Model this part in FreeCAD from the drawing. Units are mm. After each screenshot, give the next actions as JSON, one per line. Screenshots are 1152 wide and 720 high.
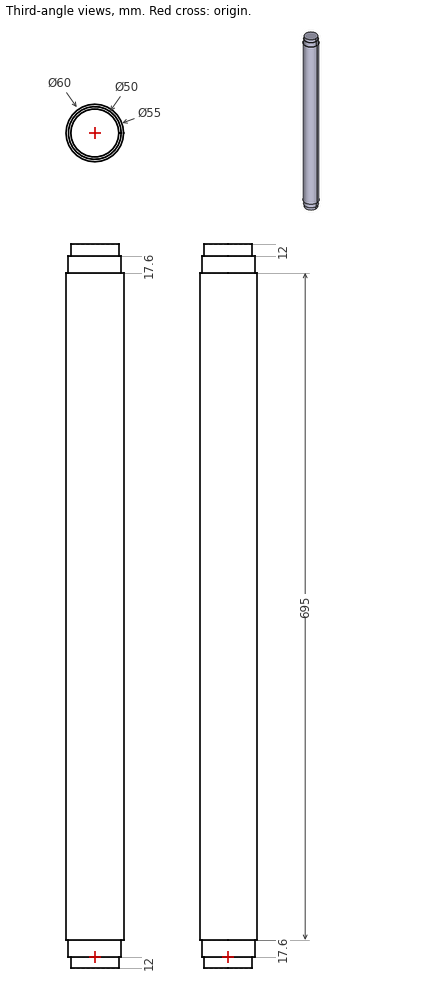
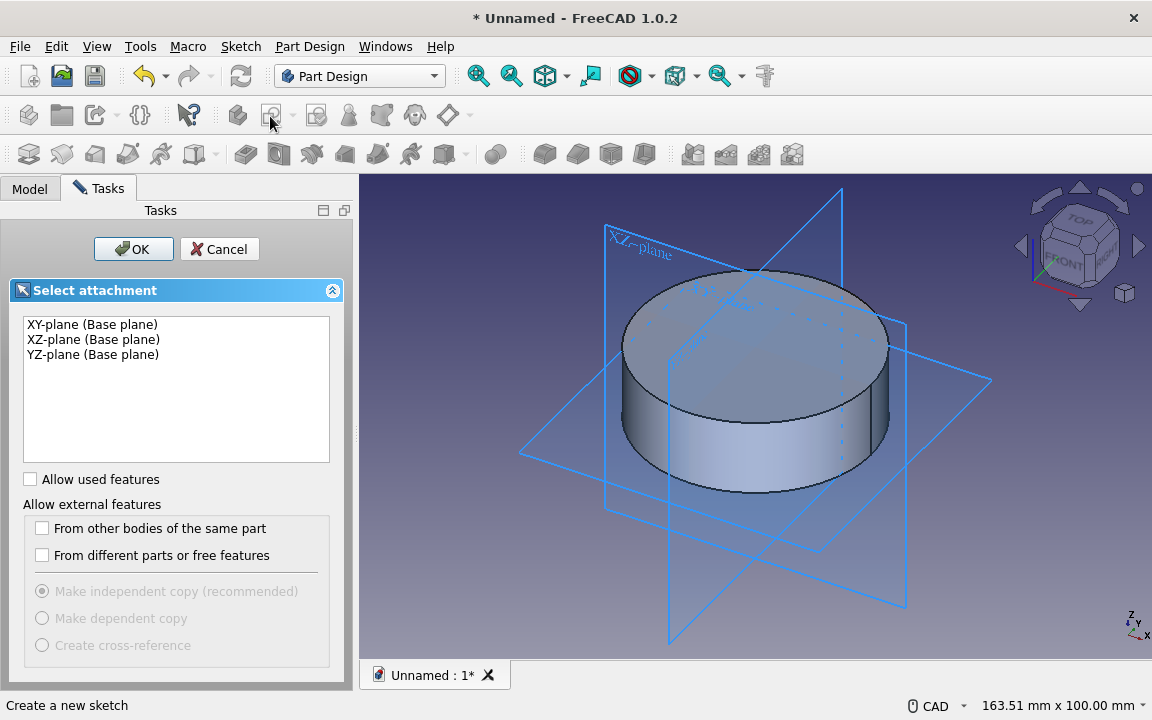
{"action": "left_click", "coordinate": [84, 324]}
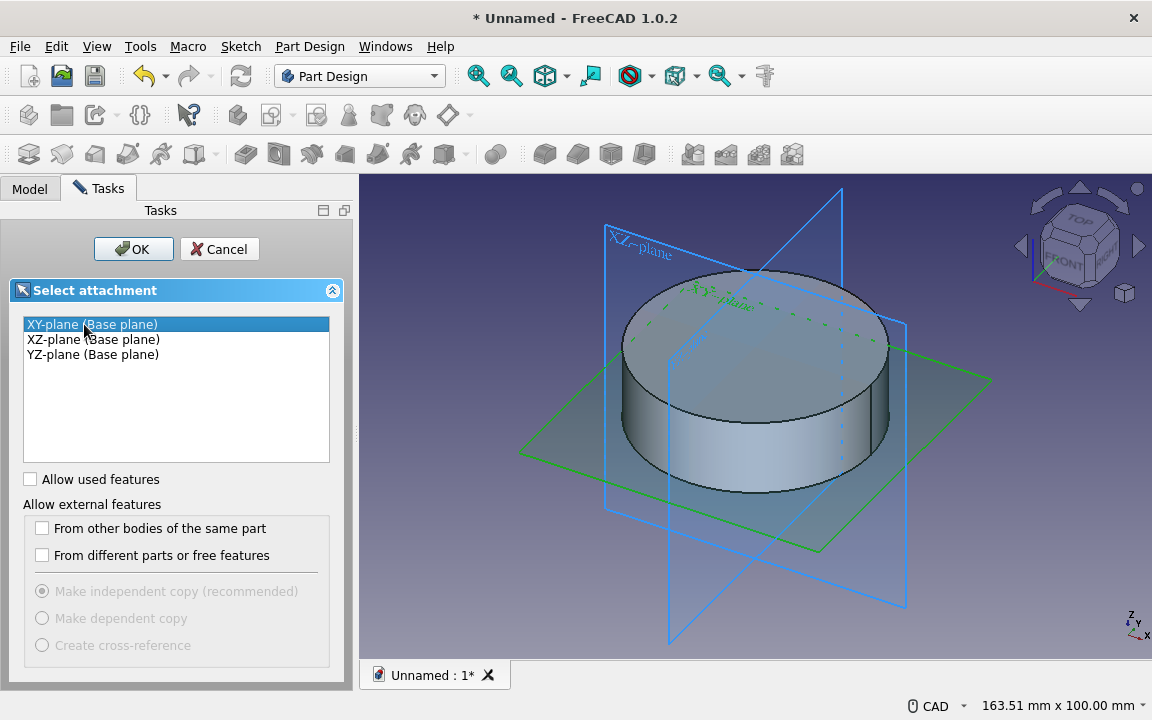
{"action": "left_click", "coordinate": [134, 249]}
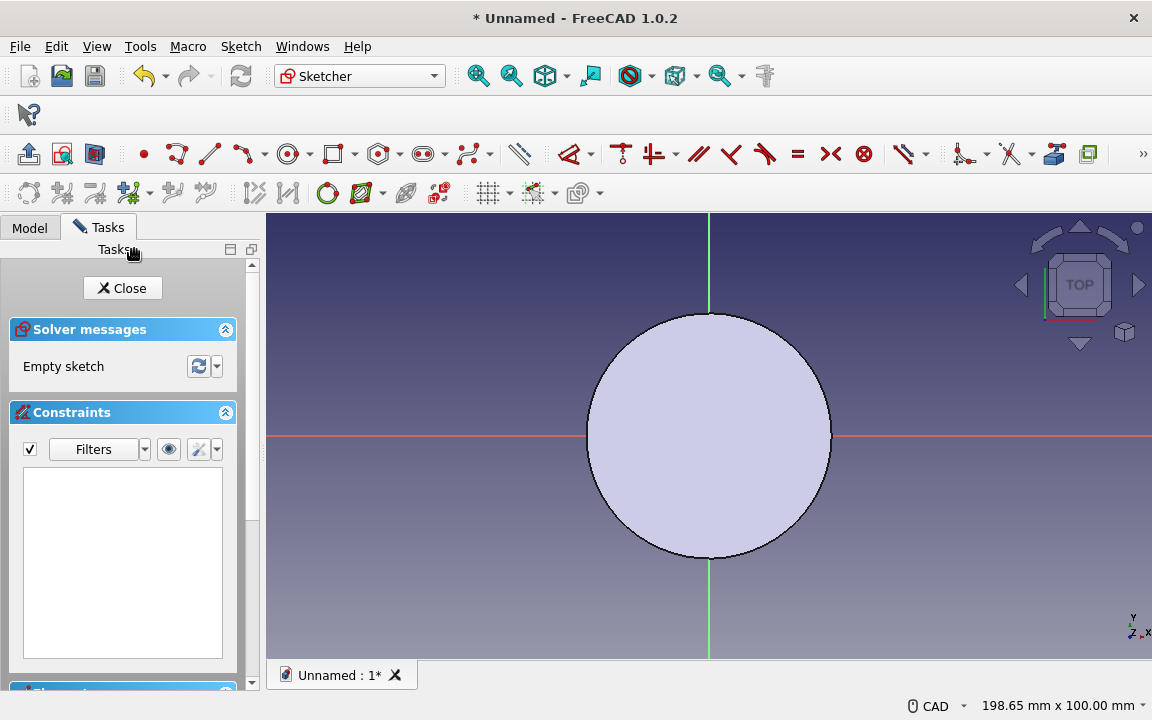
{"action": "left_click", "coordinate": [95, 154]}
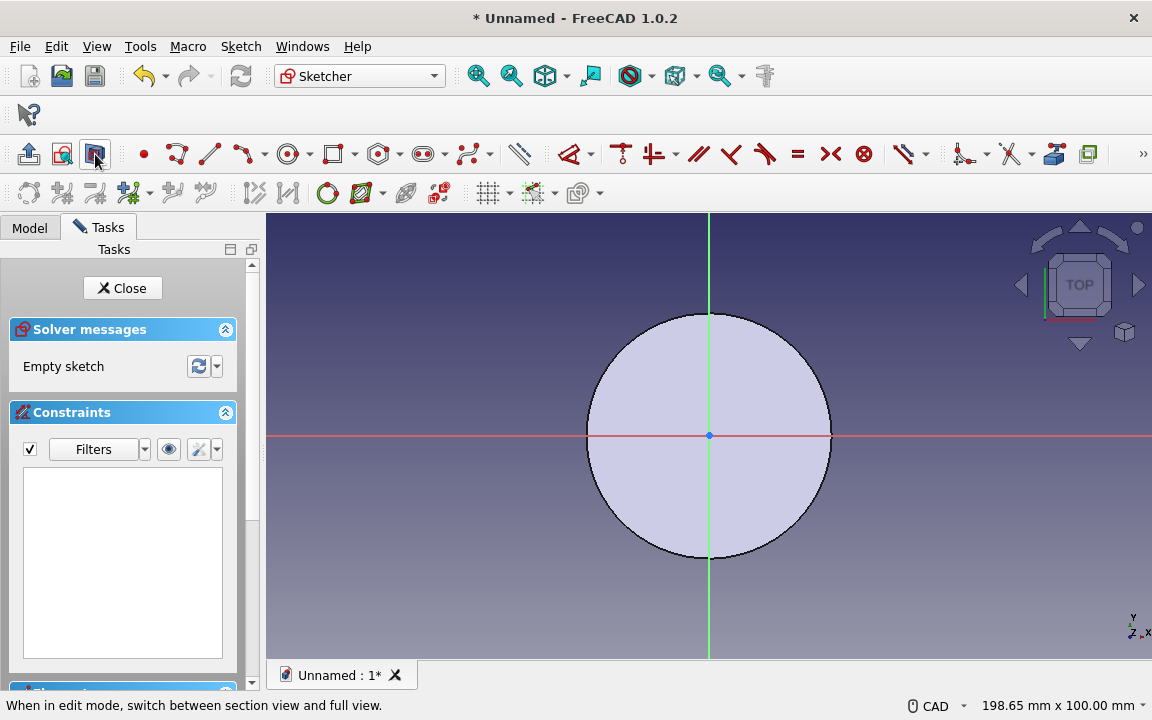
{"action": "left_click", "coordinate": [288, 154]}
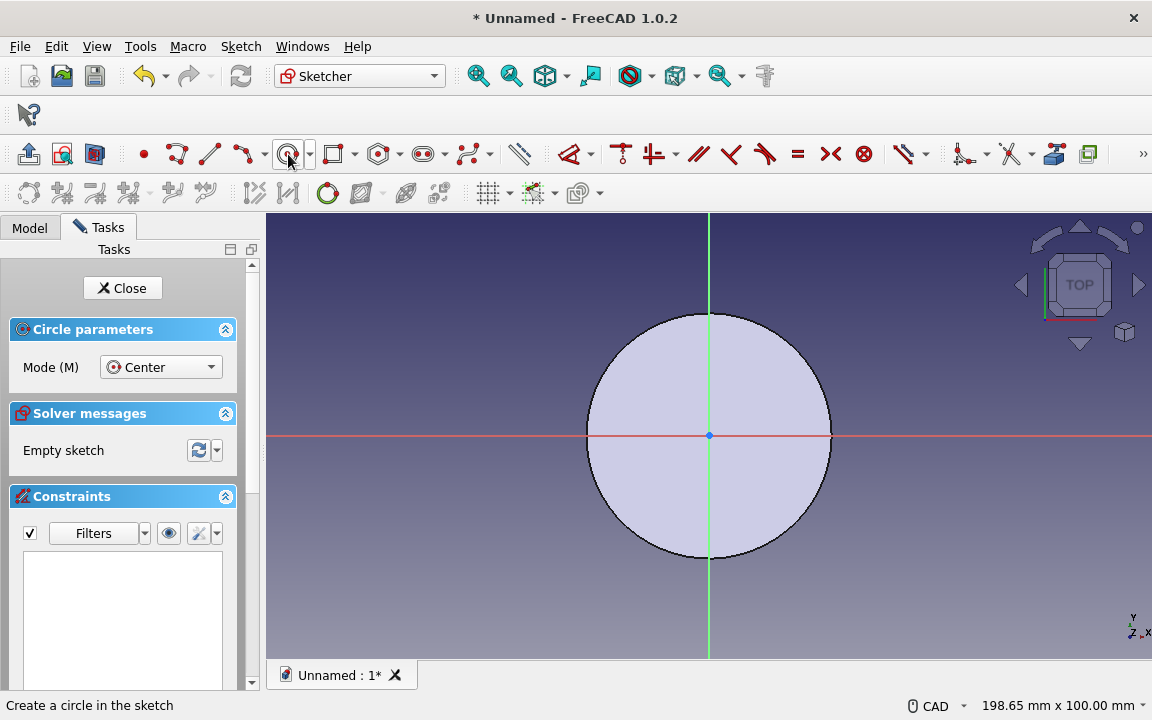
{"action": "left_click", "coordinate": [709, 436]}
{"action": "mouse_move", "coordinate": [788, 357]}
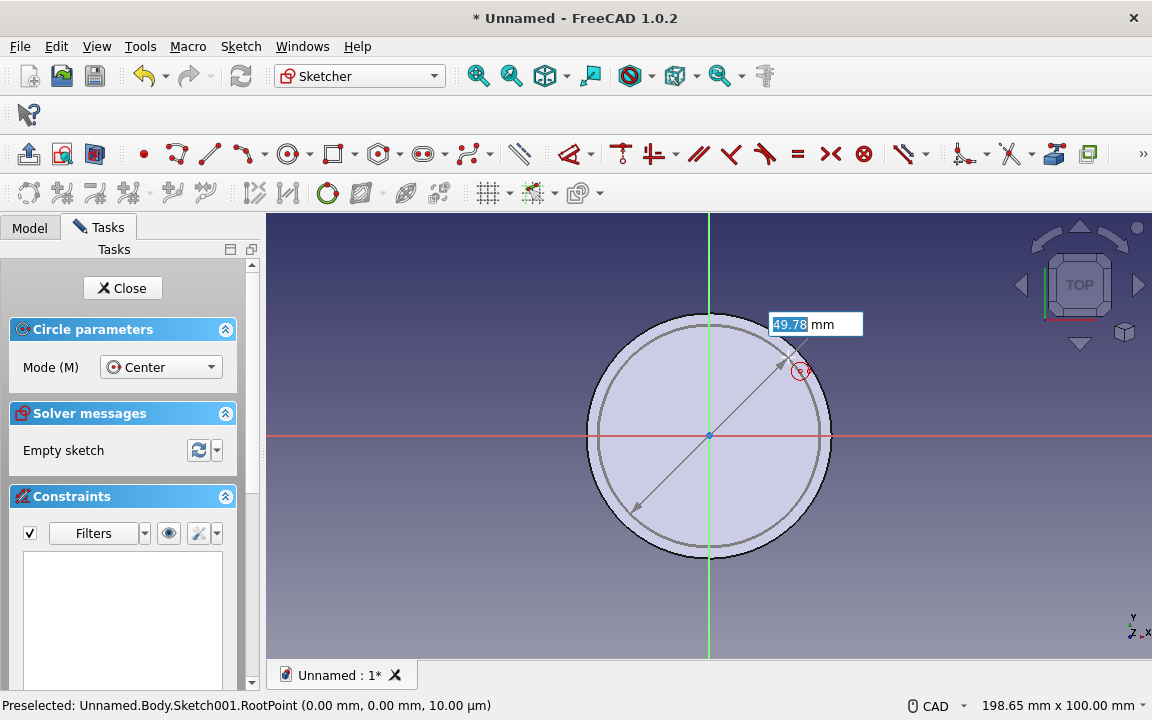
{"action": "type", "text": "50"}
{"action": "key", "text": "Return"}
{"action": "key", "text": "Escape"}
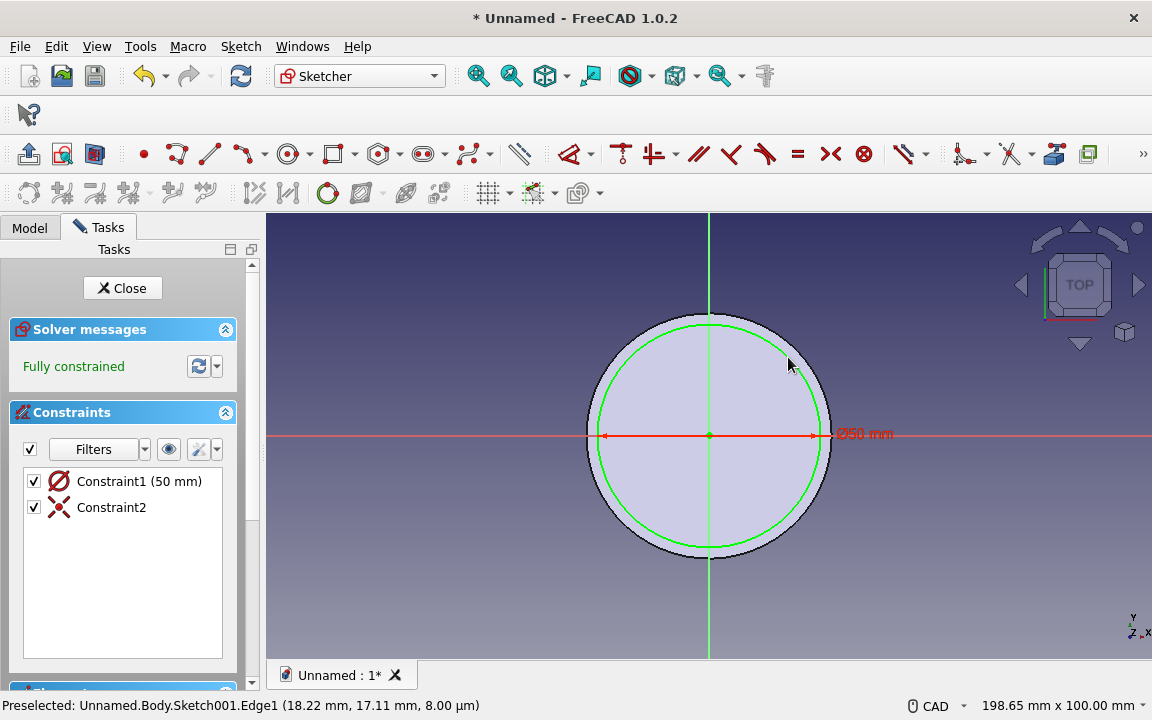
{"action": "left_click", "coordinate": [123, 288]}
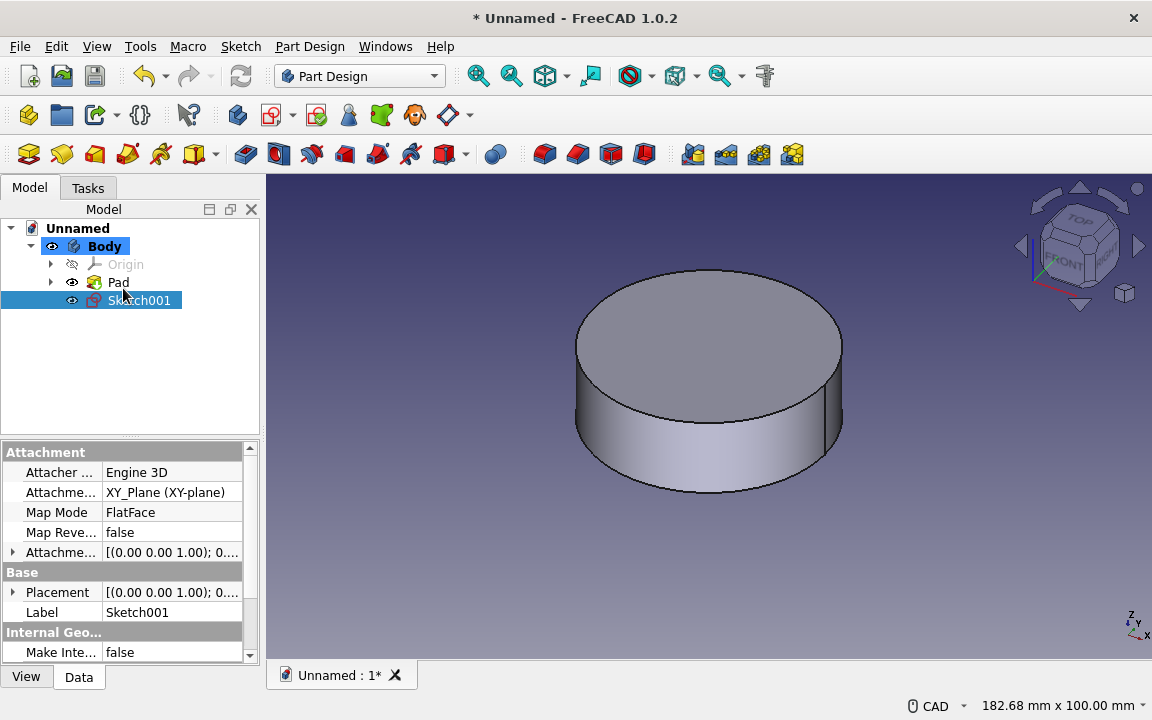
{"action": "left_click", "coordinate": [29, 154]}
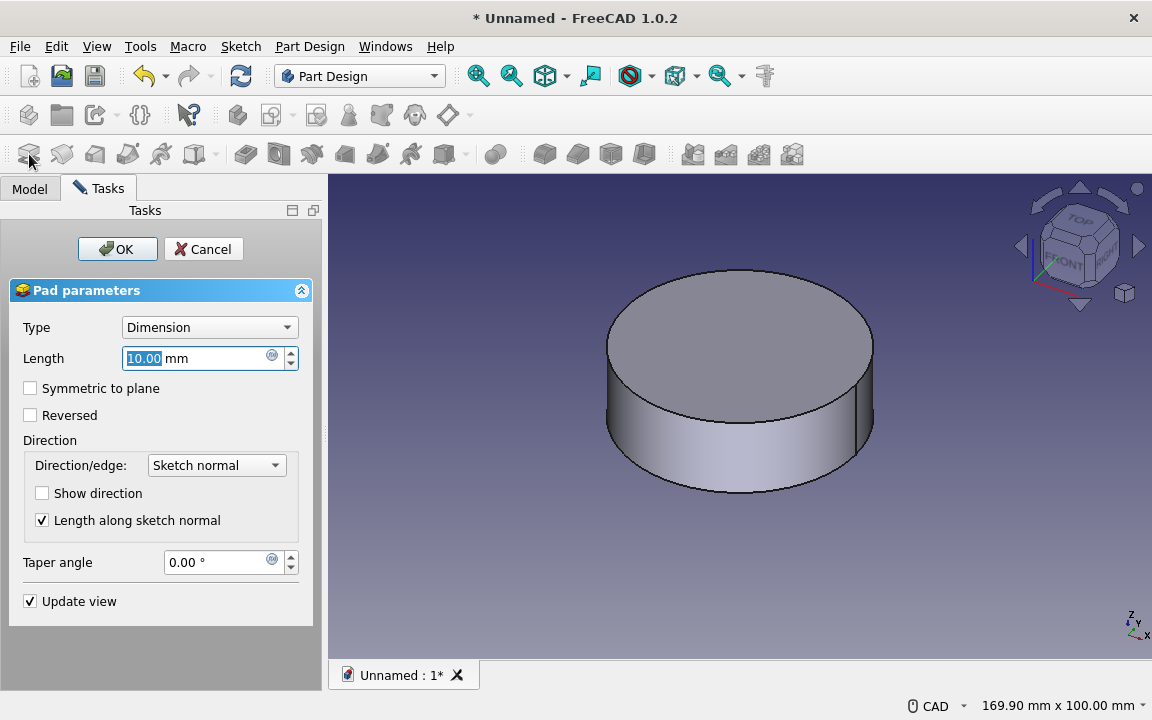
{"action": "type", "text": "12"}
{"action": "key", "text": "Tab"}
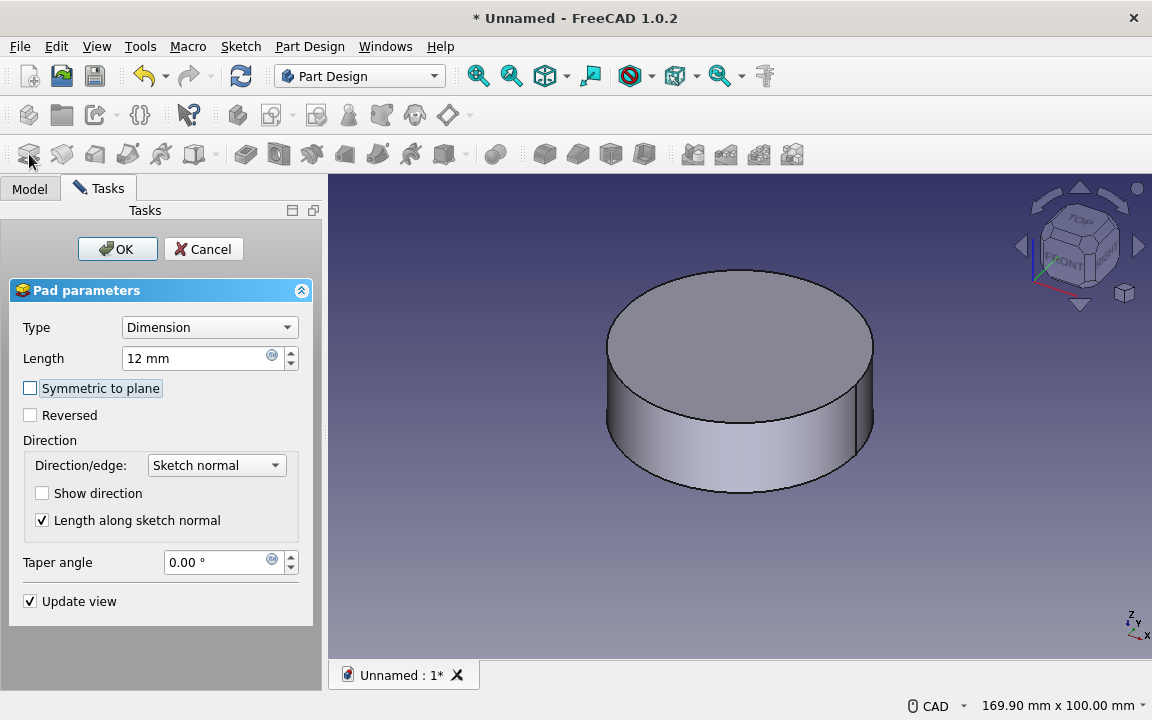
{"action": "left_click", "coordinate": [31, 415]}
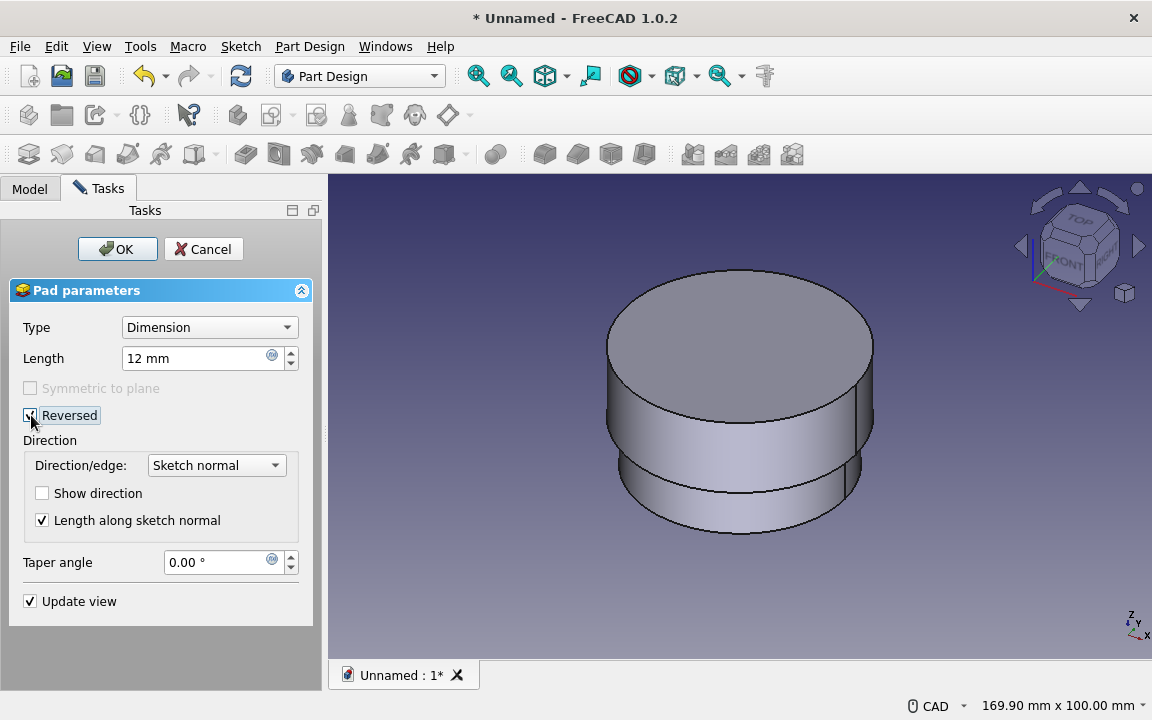
{"action": "left_click", "coordinate": [118, 249]}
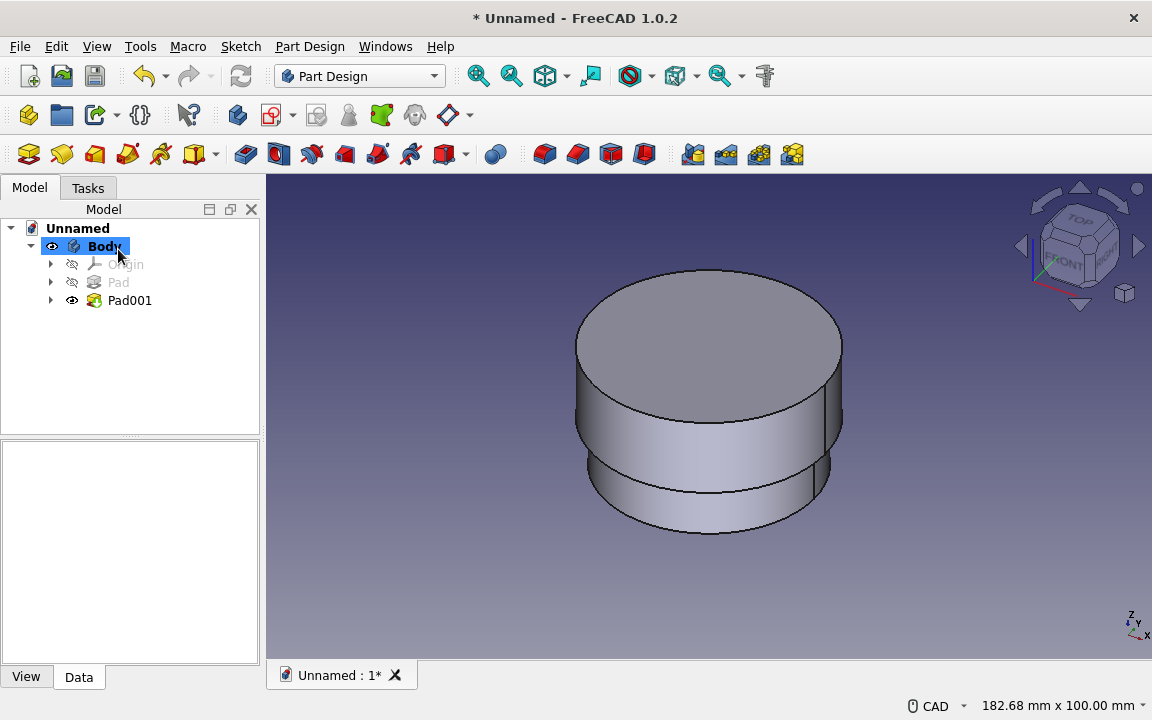
{"action": "left_click", "coordinate": [709, 346]}